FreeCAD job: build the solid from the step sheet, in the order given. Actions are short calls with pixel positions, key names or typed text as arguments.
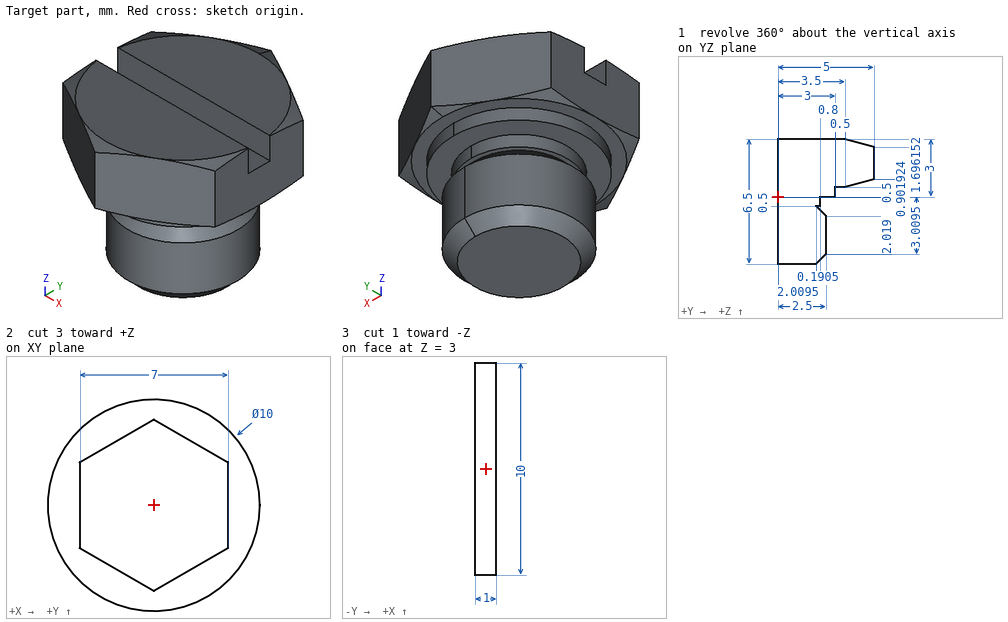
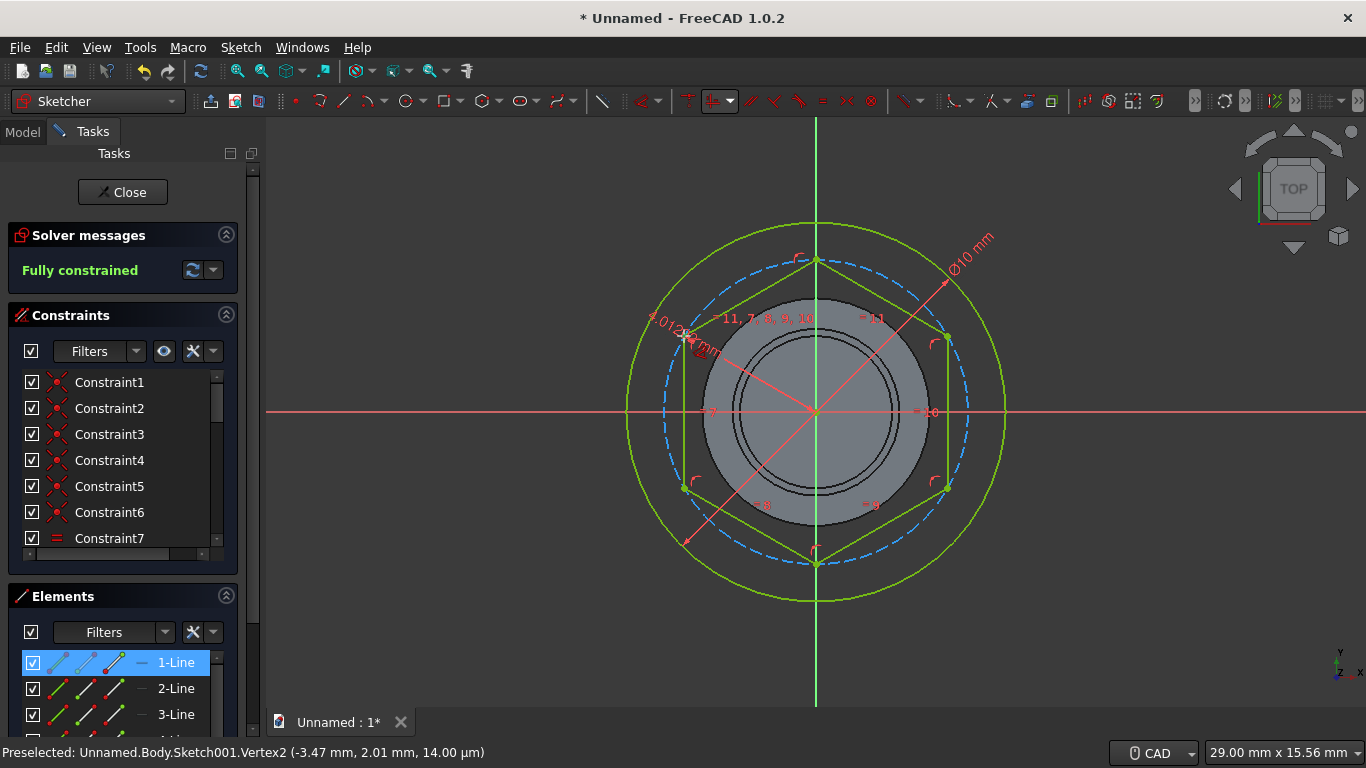
click(948, 488)
click(755, 570)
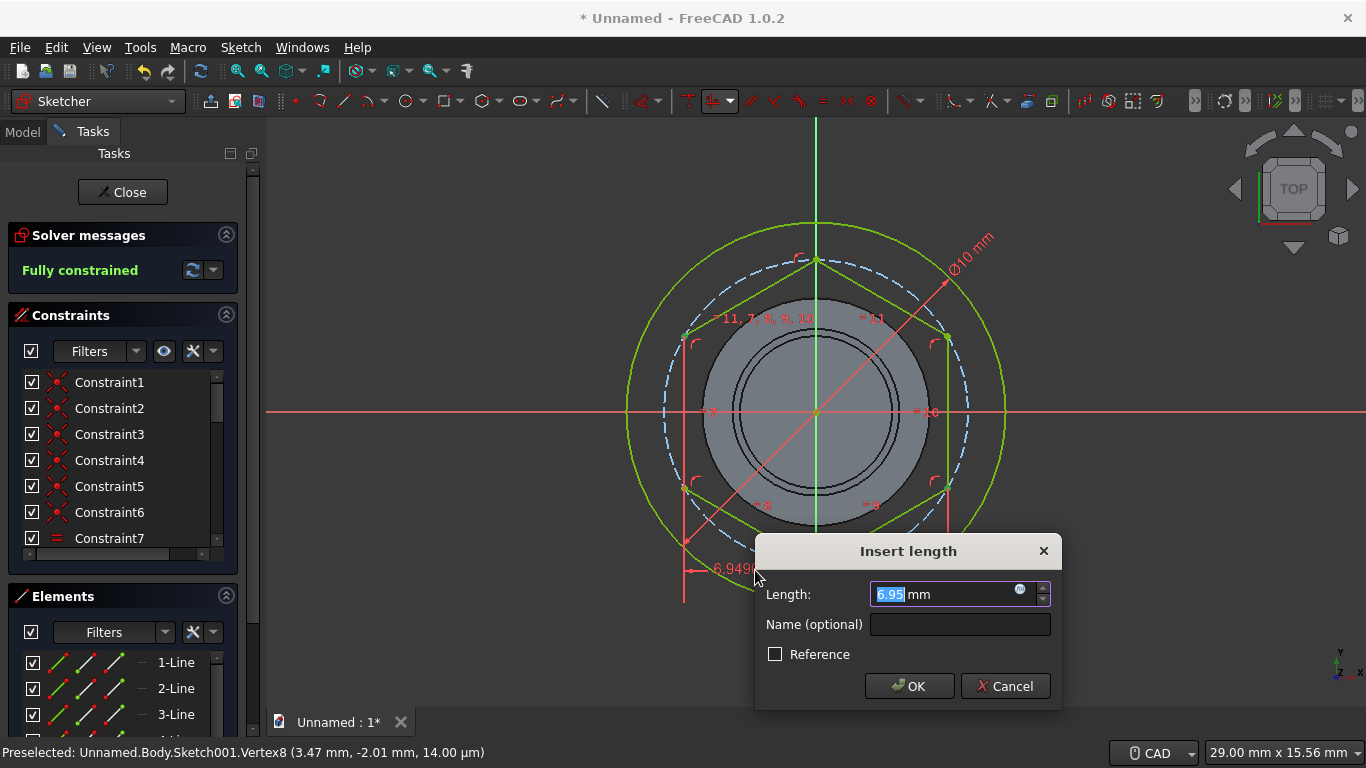
text(7)
key(Return)
key(Escape)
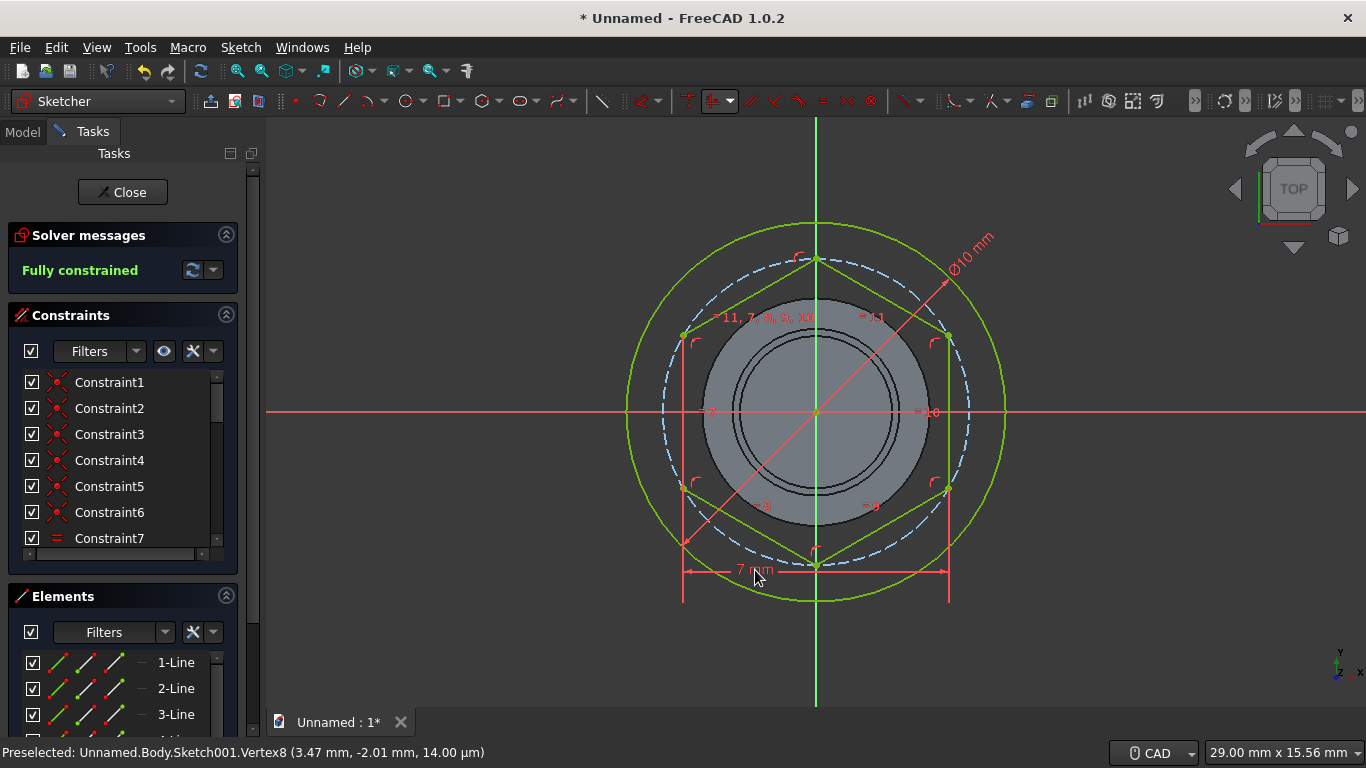
click(123, 192)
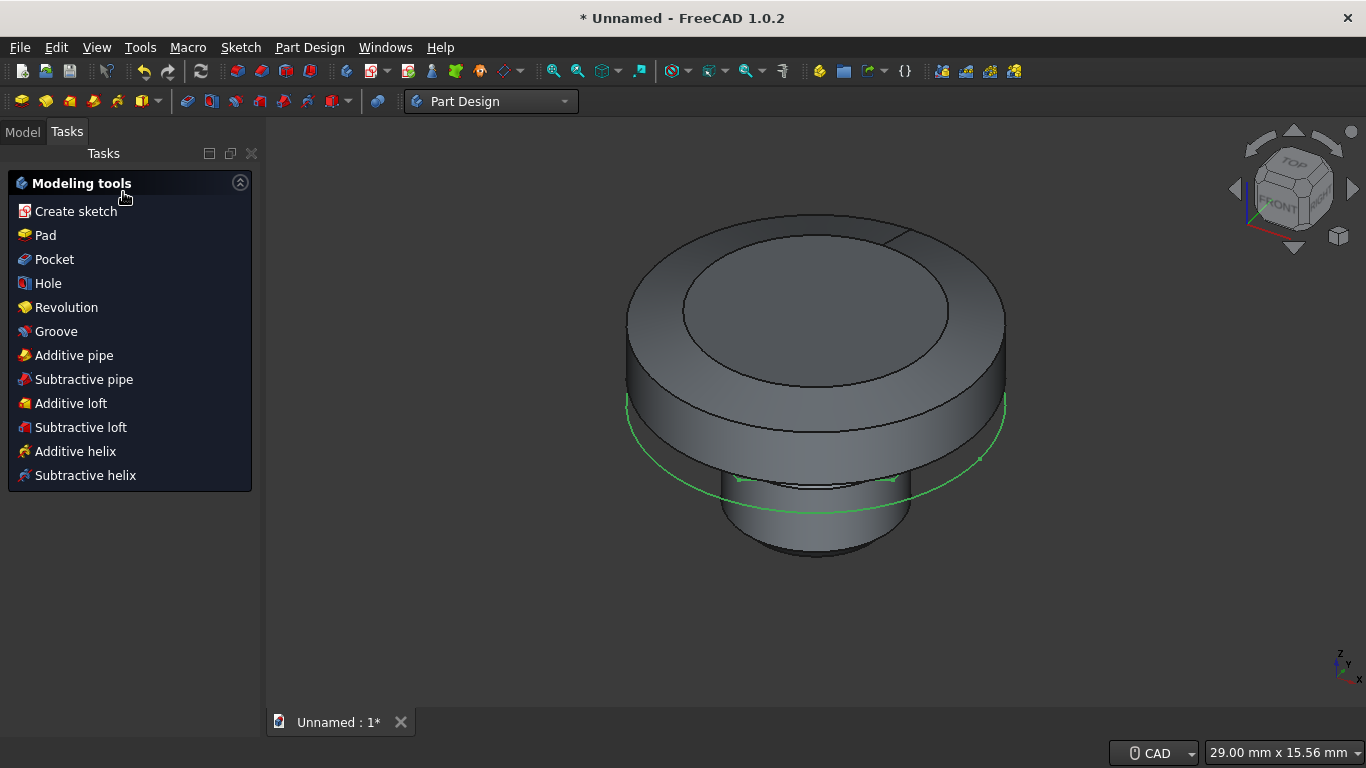
click(188, 102)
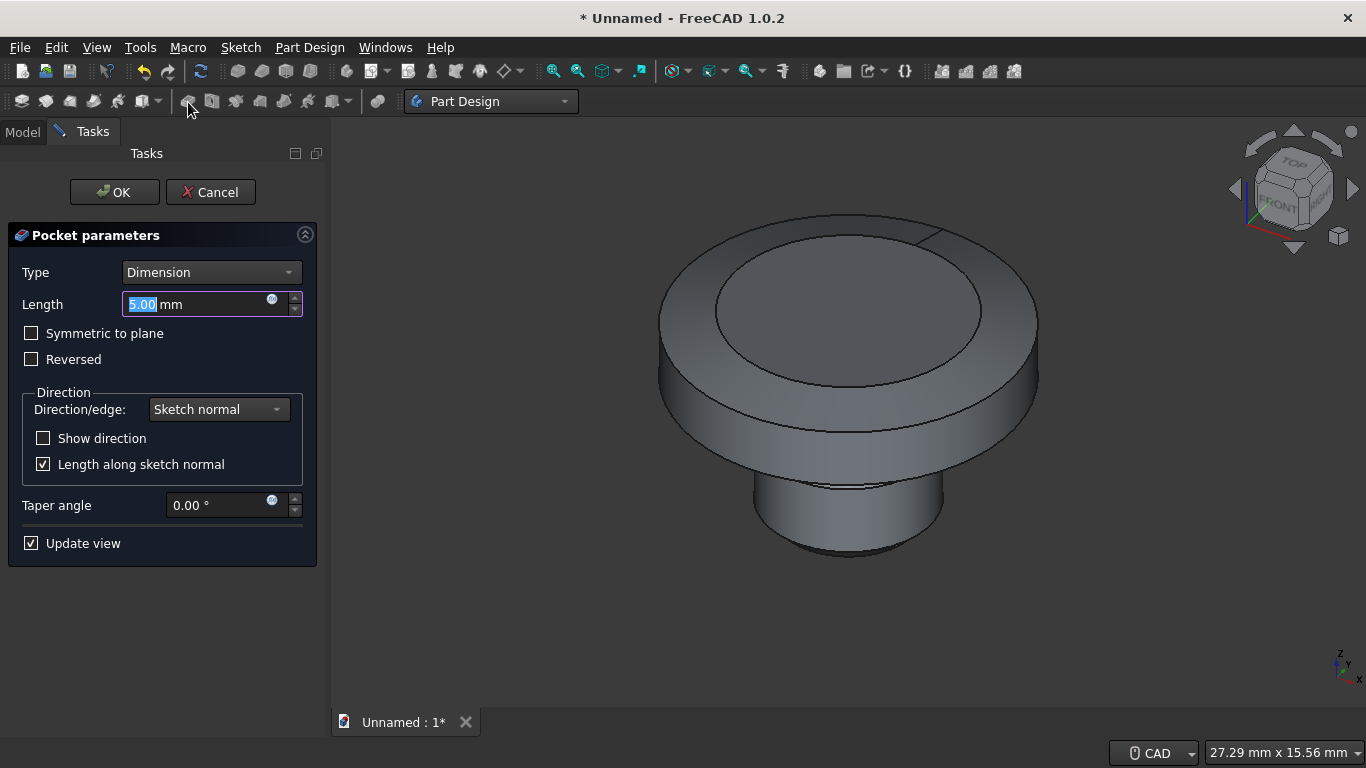
text(3)
key(Tab)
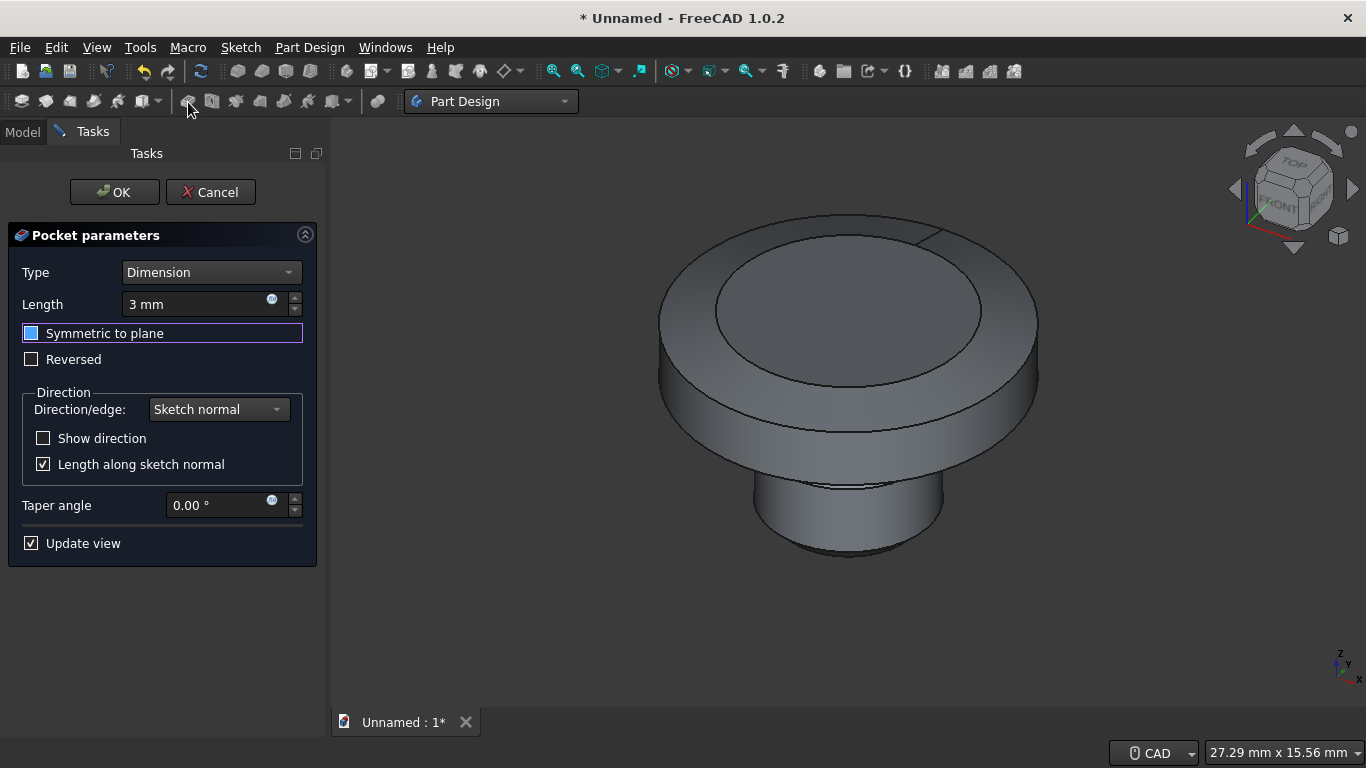
click(30, 359)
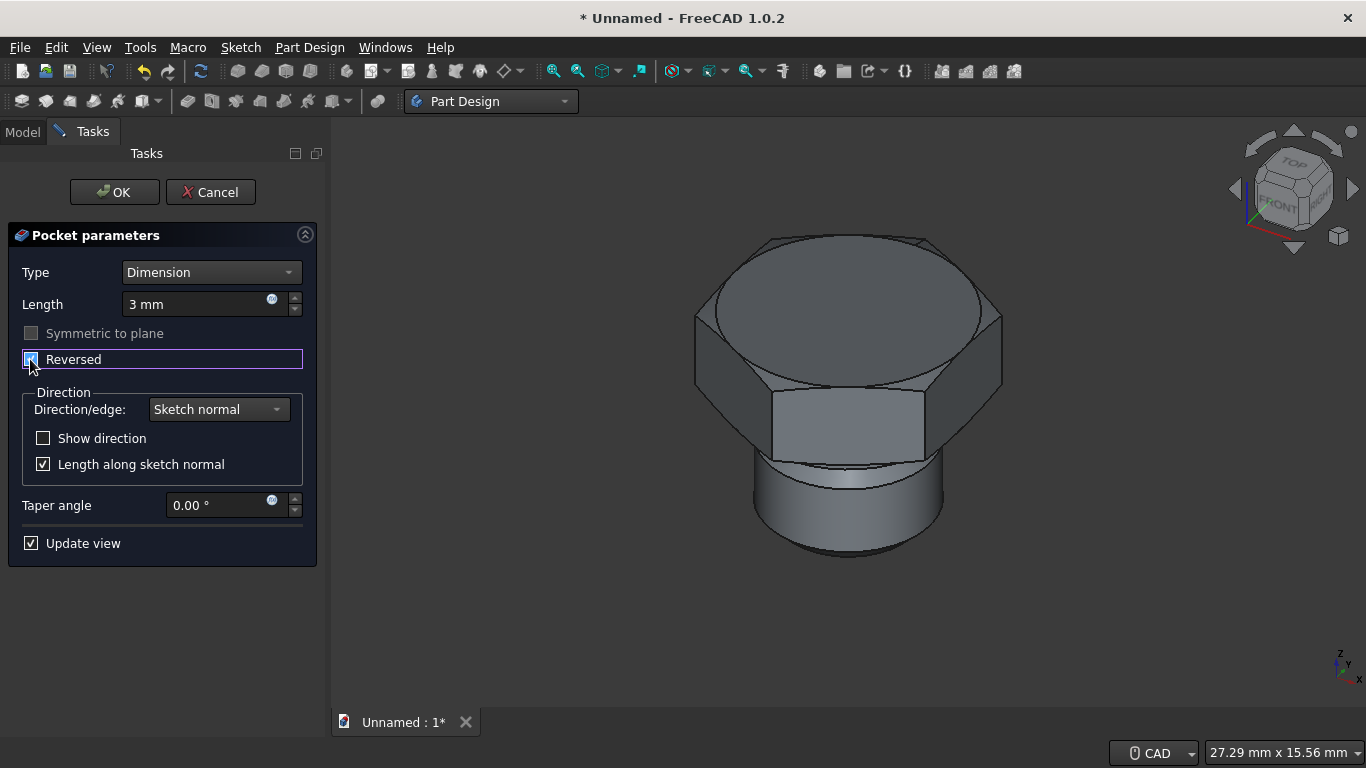
click(115, 192)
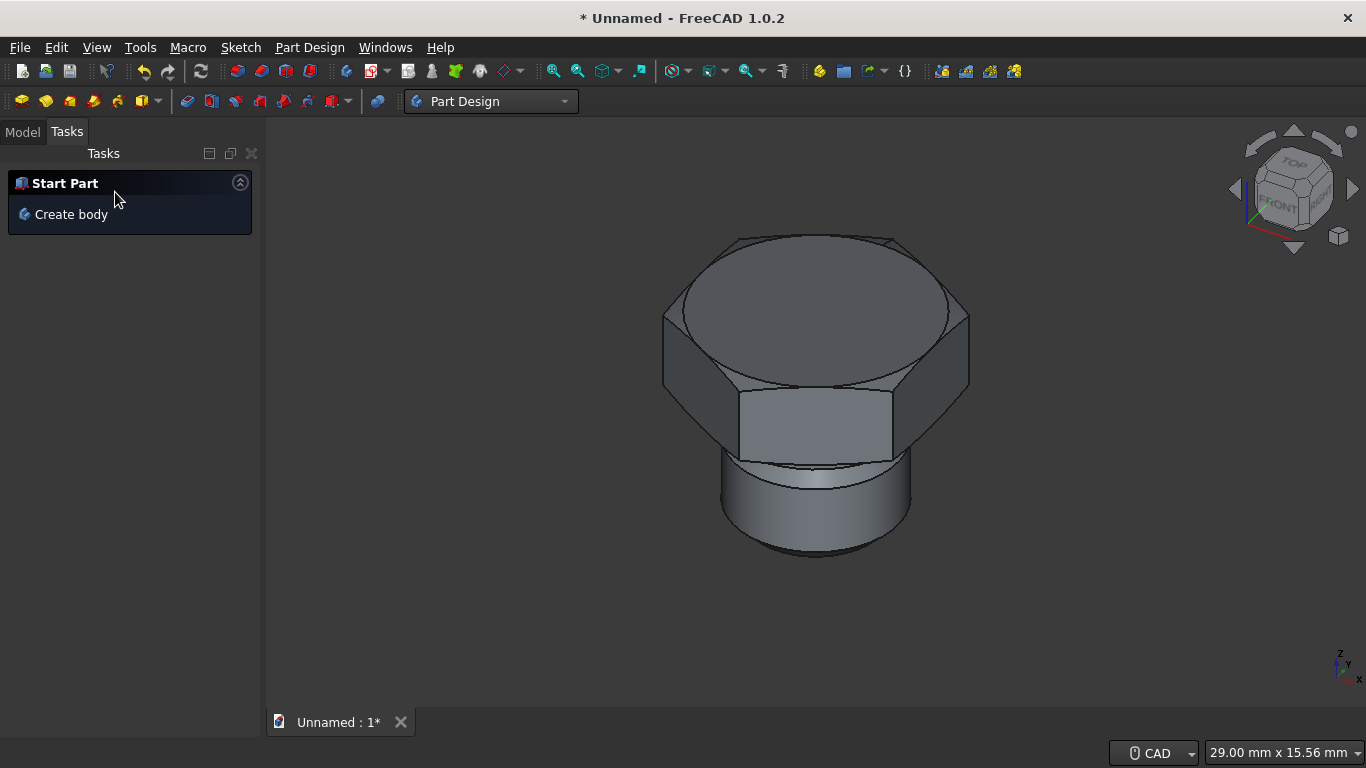
click(816, 310)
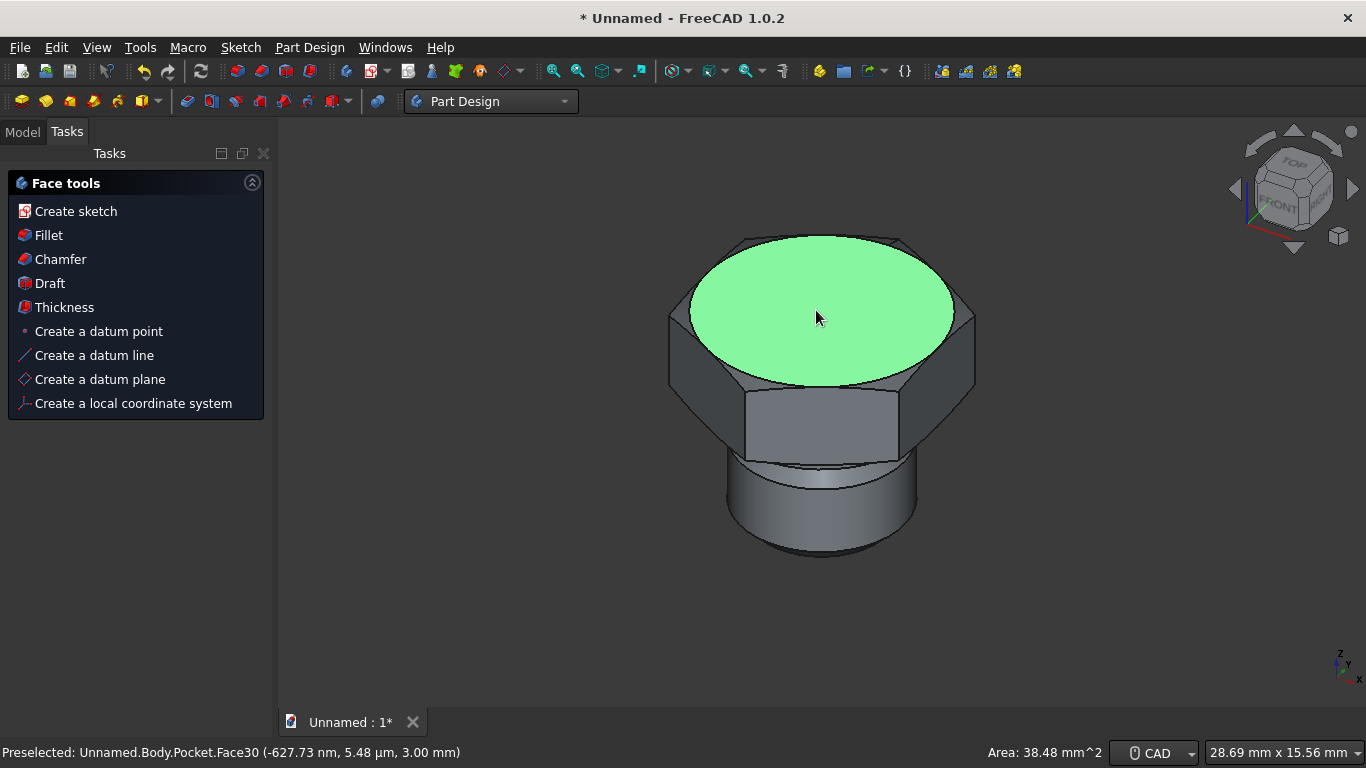
click(372, 72)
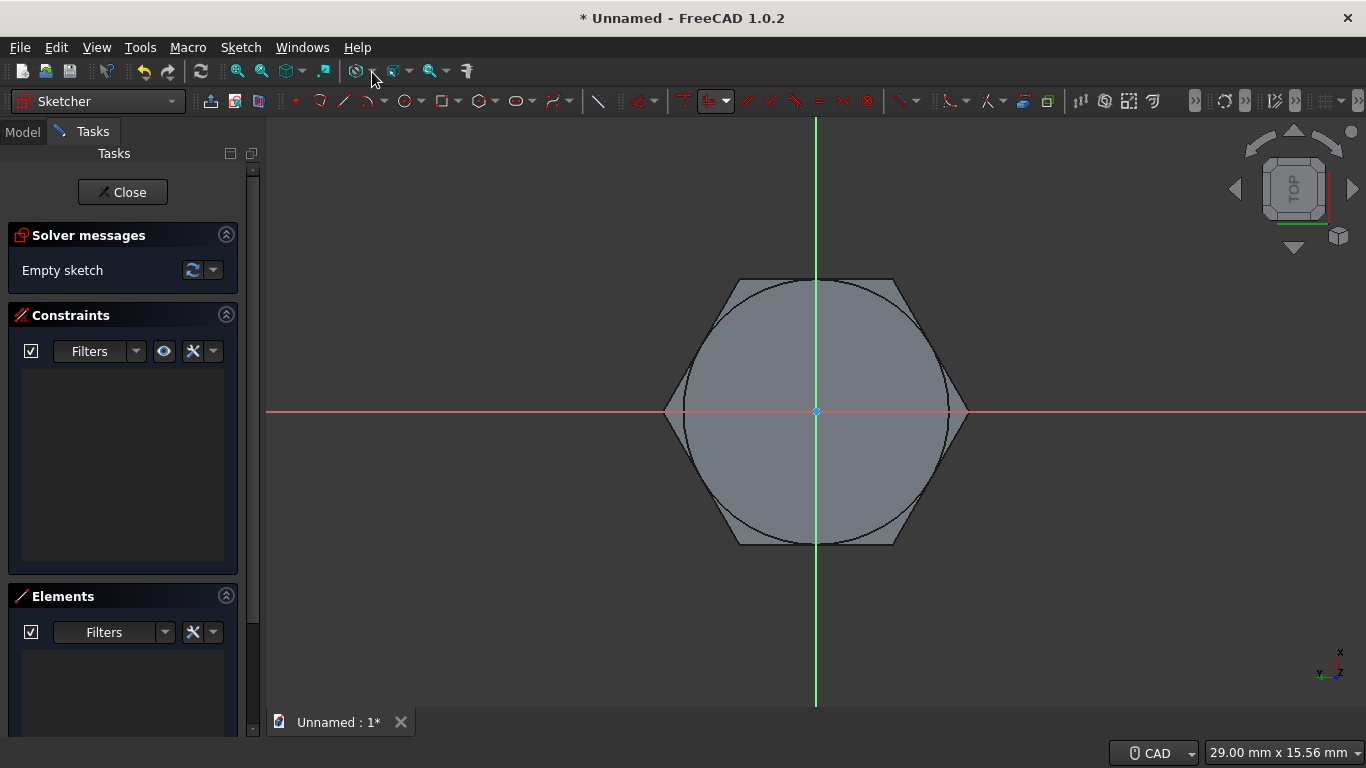
click(460, 102)